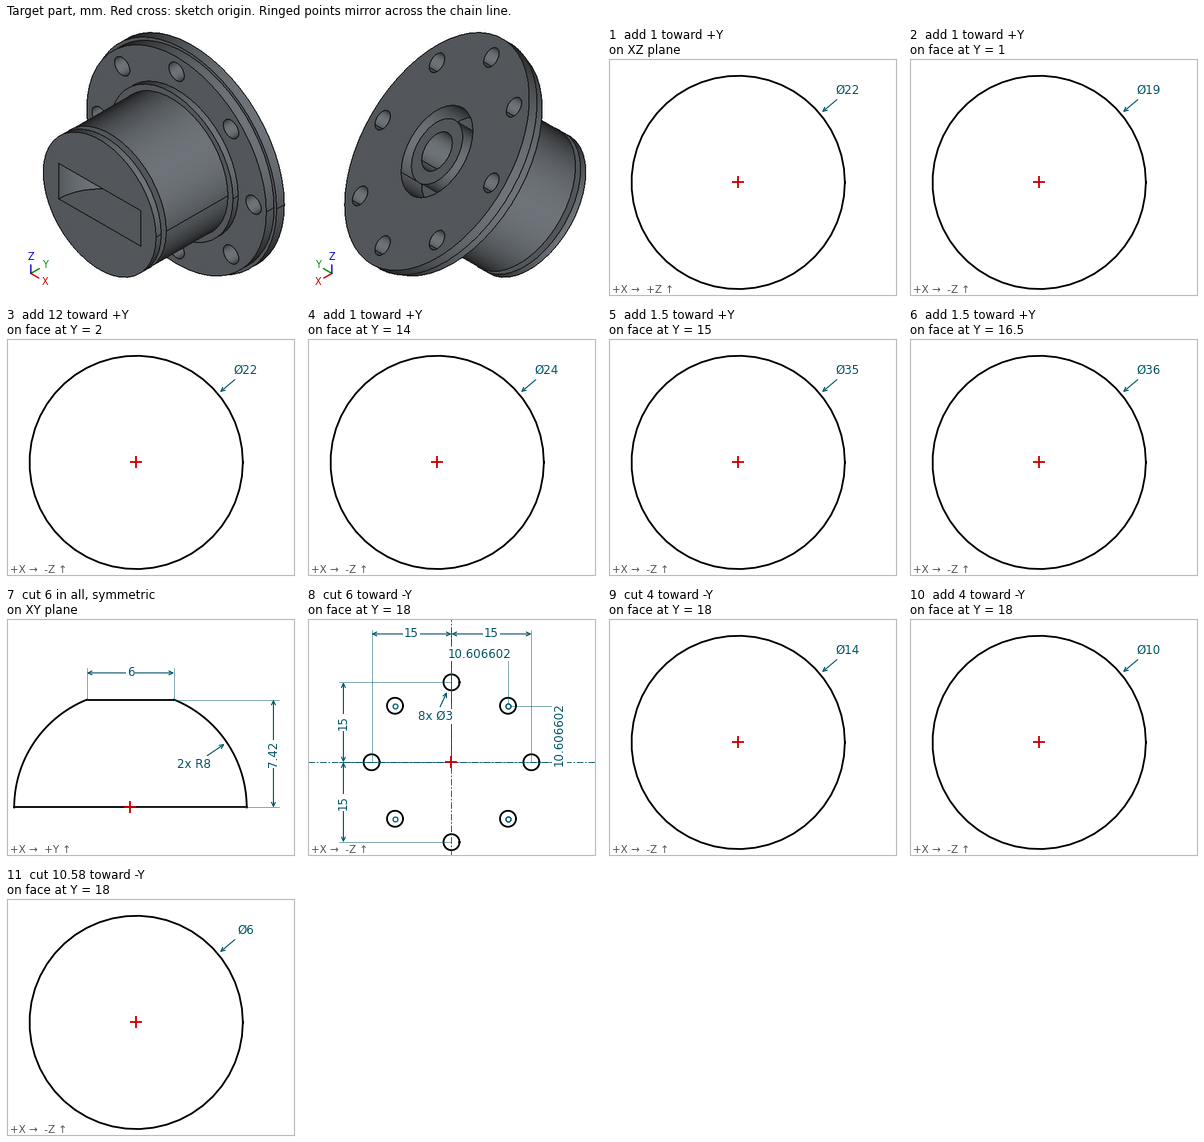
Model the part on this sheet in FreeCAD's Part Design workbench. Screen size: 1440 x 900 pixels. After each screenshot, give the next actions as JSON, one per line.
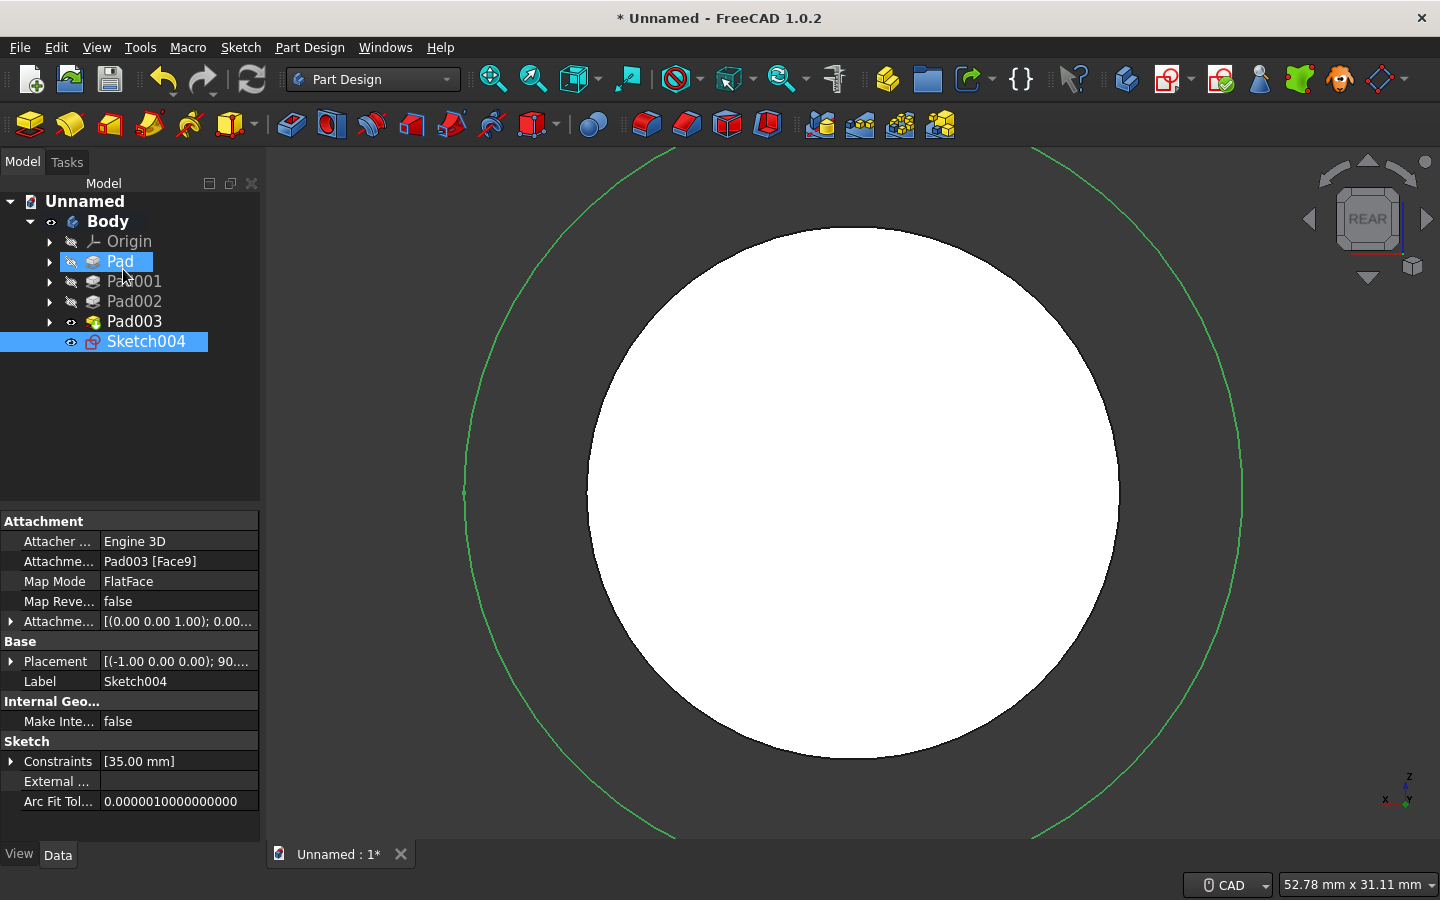
{"action": "left_click", "coordinate": [30, 124]}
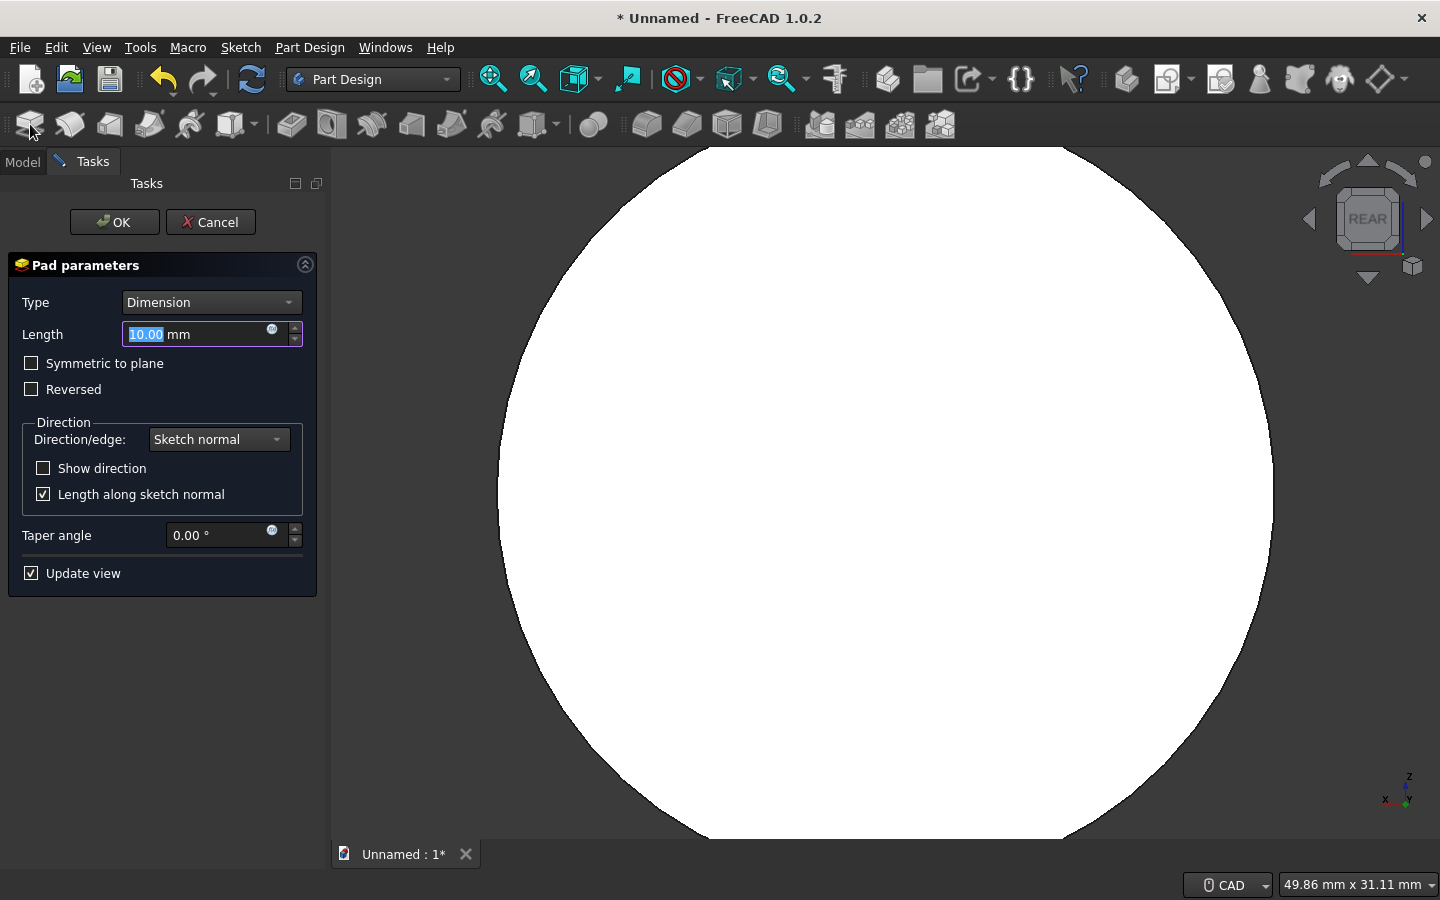
{"action": "type", "text": "1.5"}
{"action": "key", "text": "Tab"}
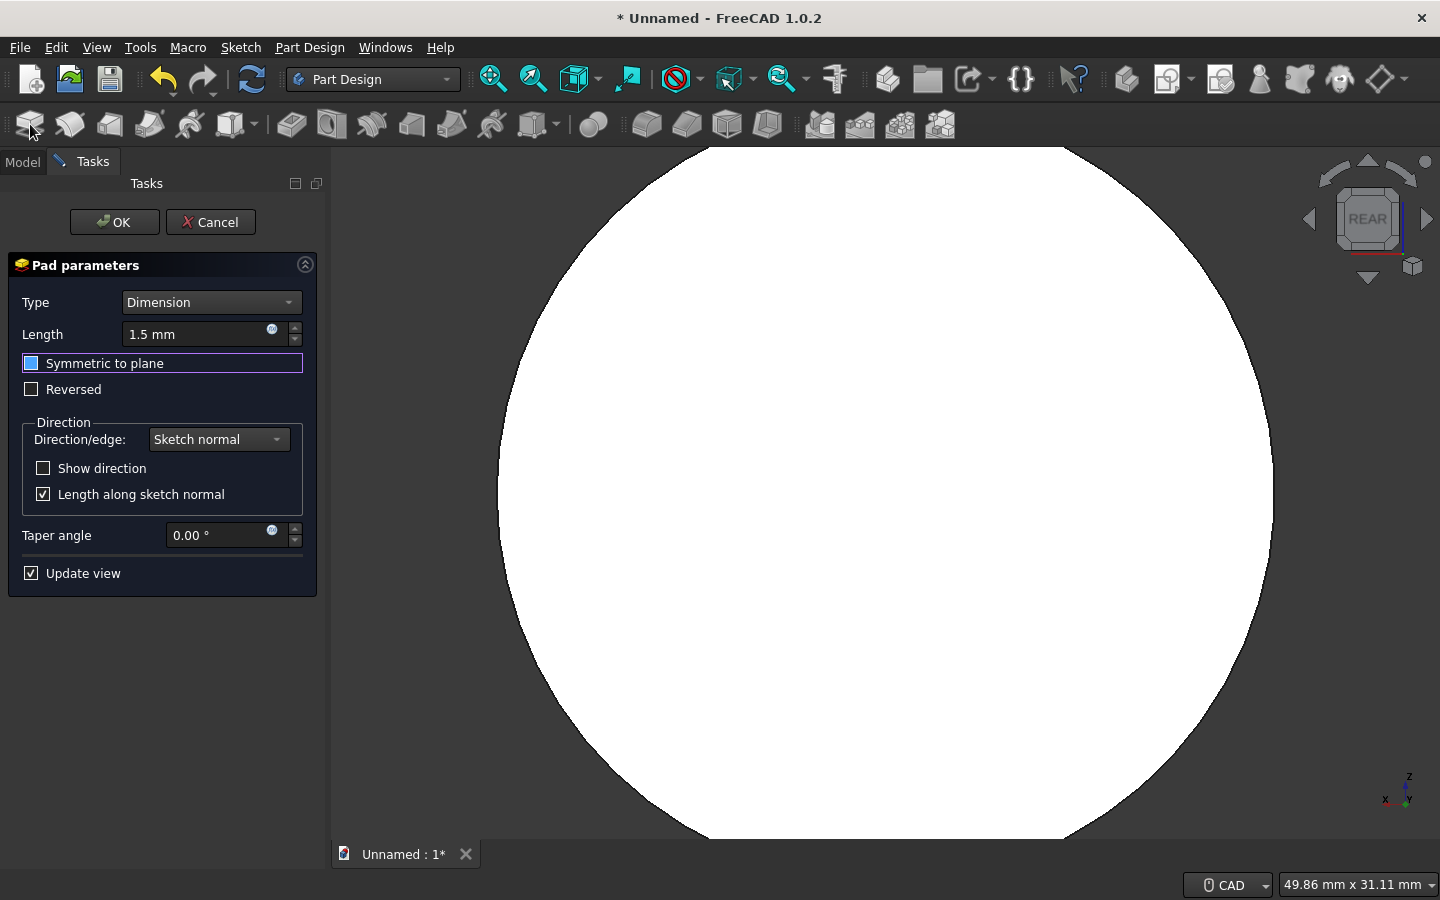
{"action": "left_click", "coordinate": [115, 222]}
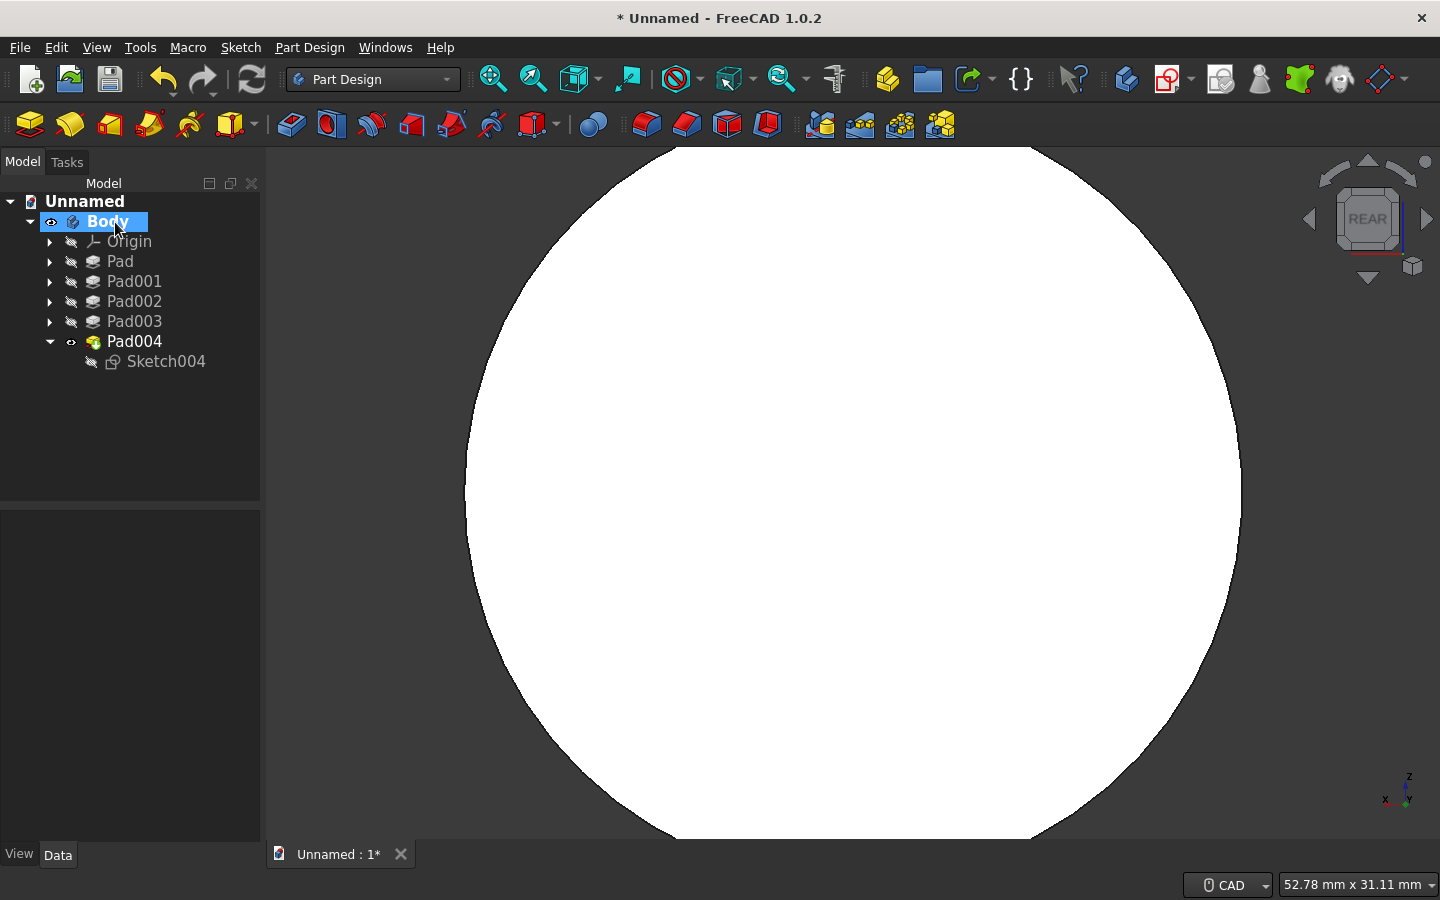
{"action": "left_click", "coordinate": [494, 80]}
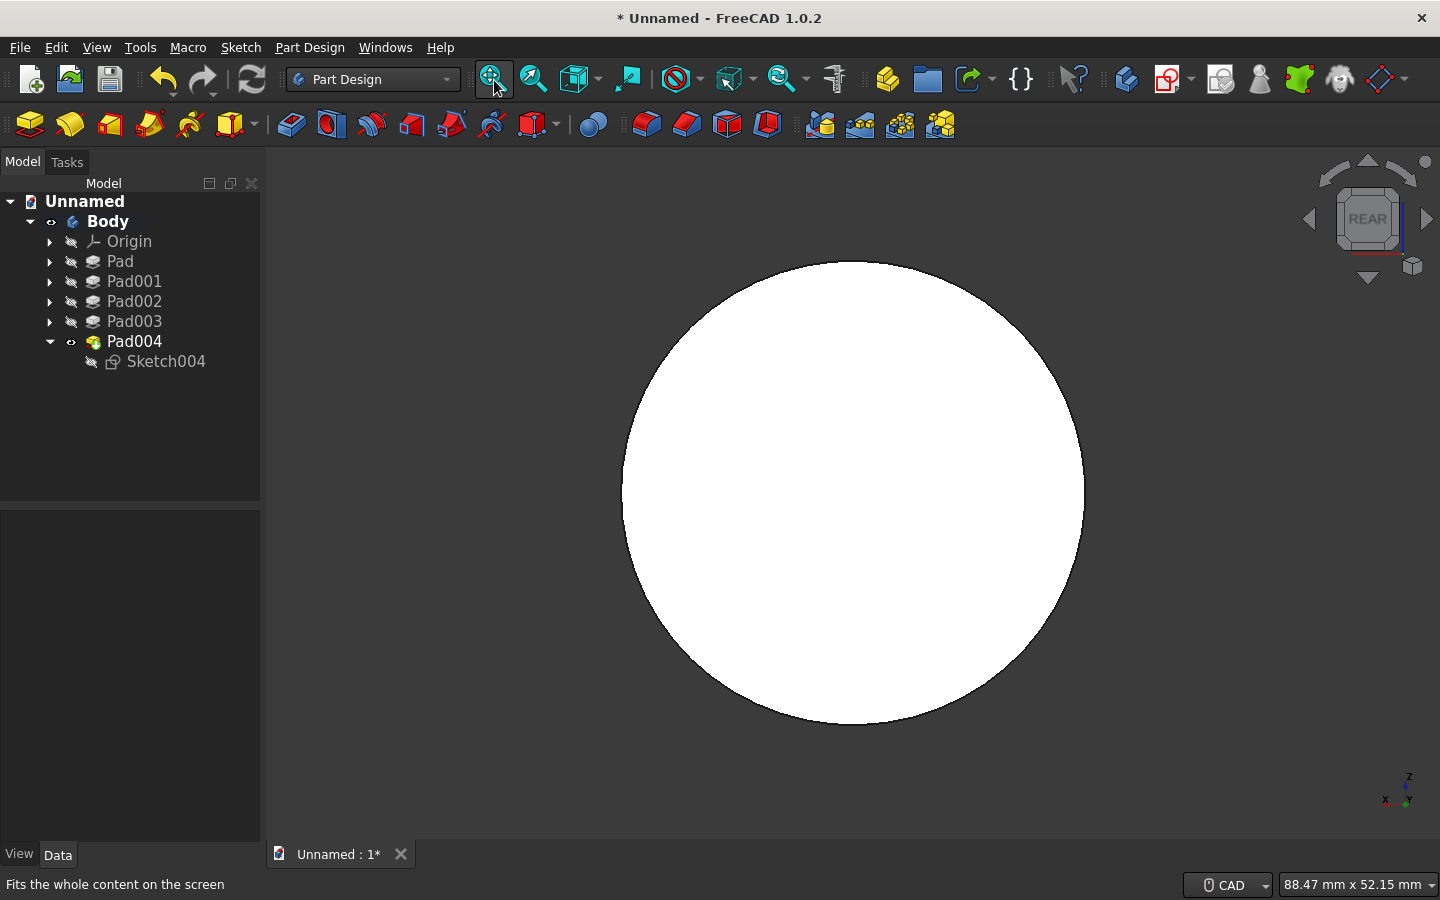
{"action": "left_click", "coordinate": [853, 492]}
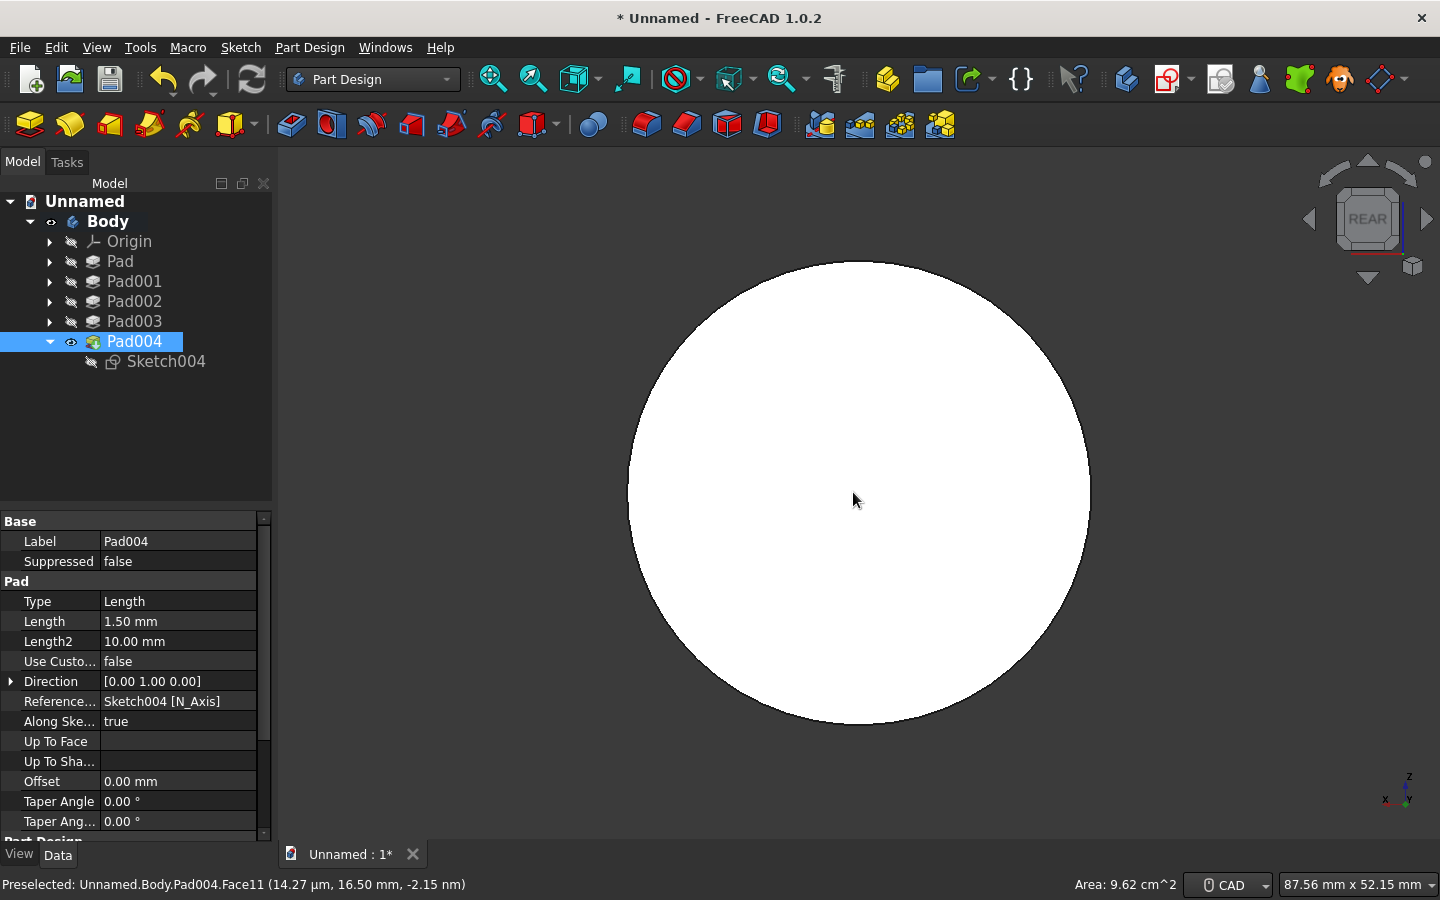
{"action": "left_click", "coordinate": [1168, 80]}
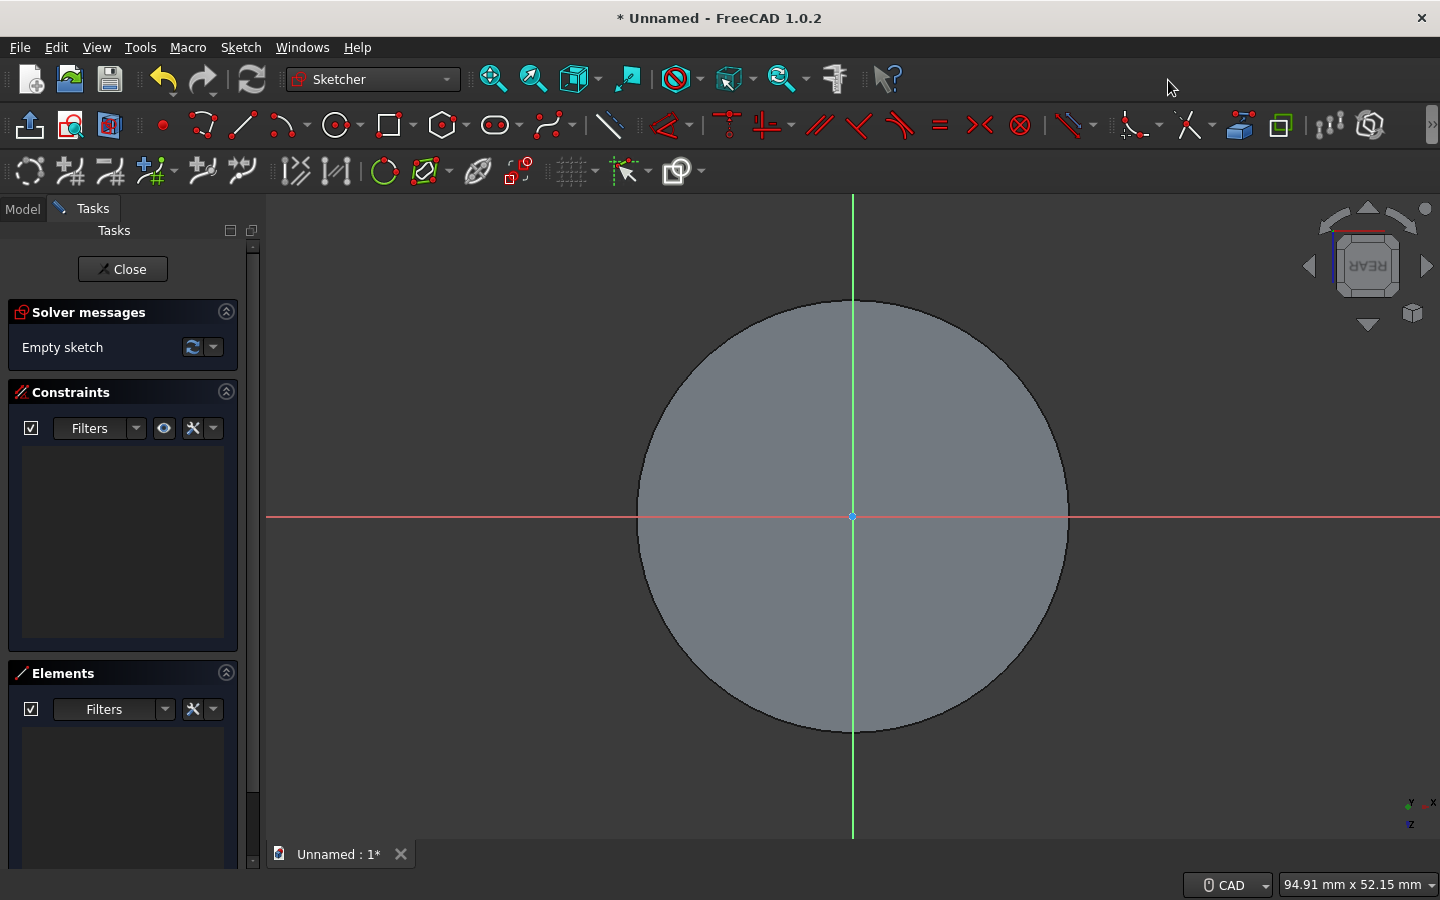
{"action": "left_click", "coordinate": [336, 126]}